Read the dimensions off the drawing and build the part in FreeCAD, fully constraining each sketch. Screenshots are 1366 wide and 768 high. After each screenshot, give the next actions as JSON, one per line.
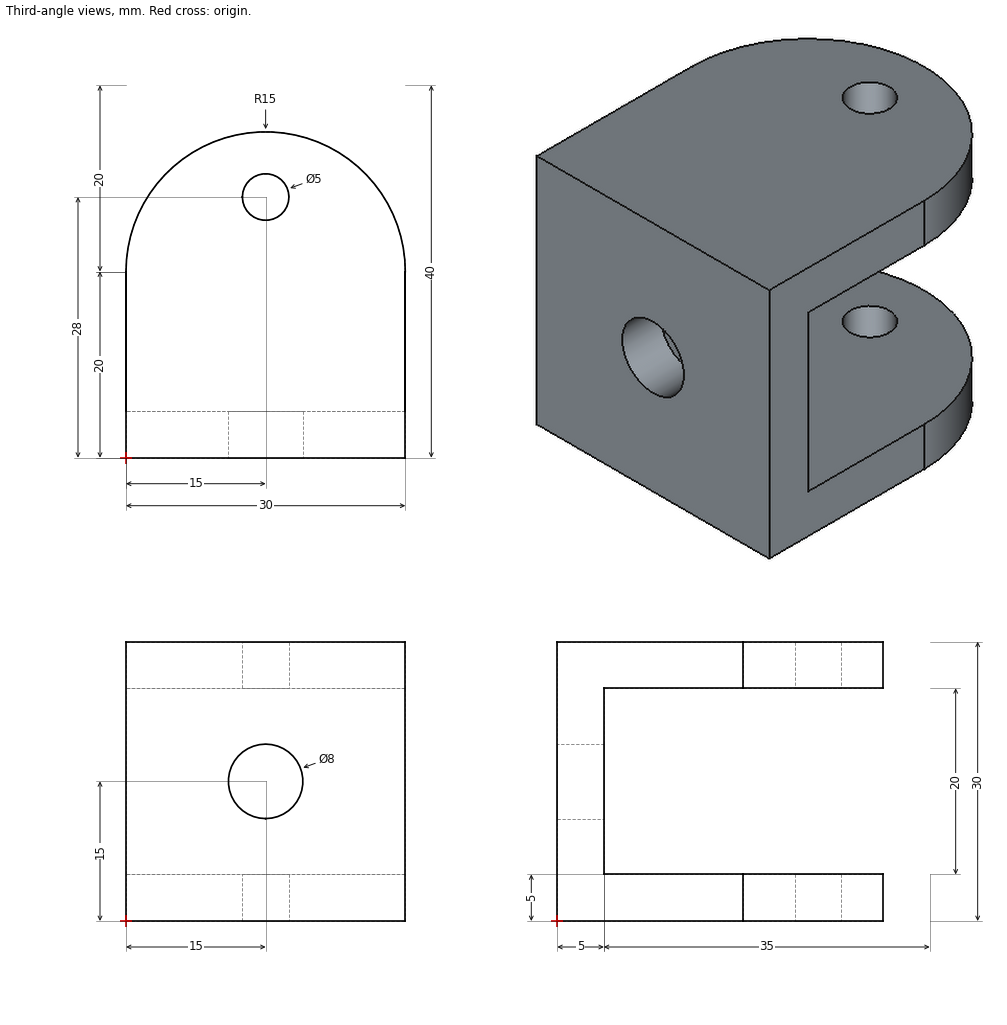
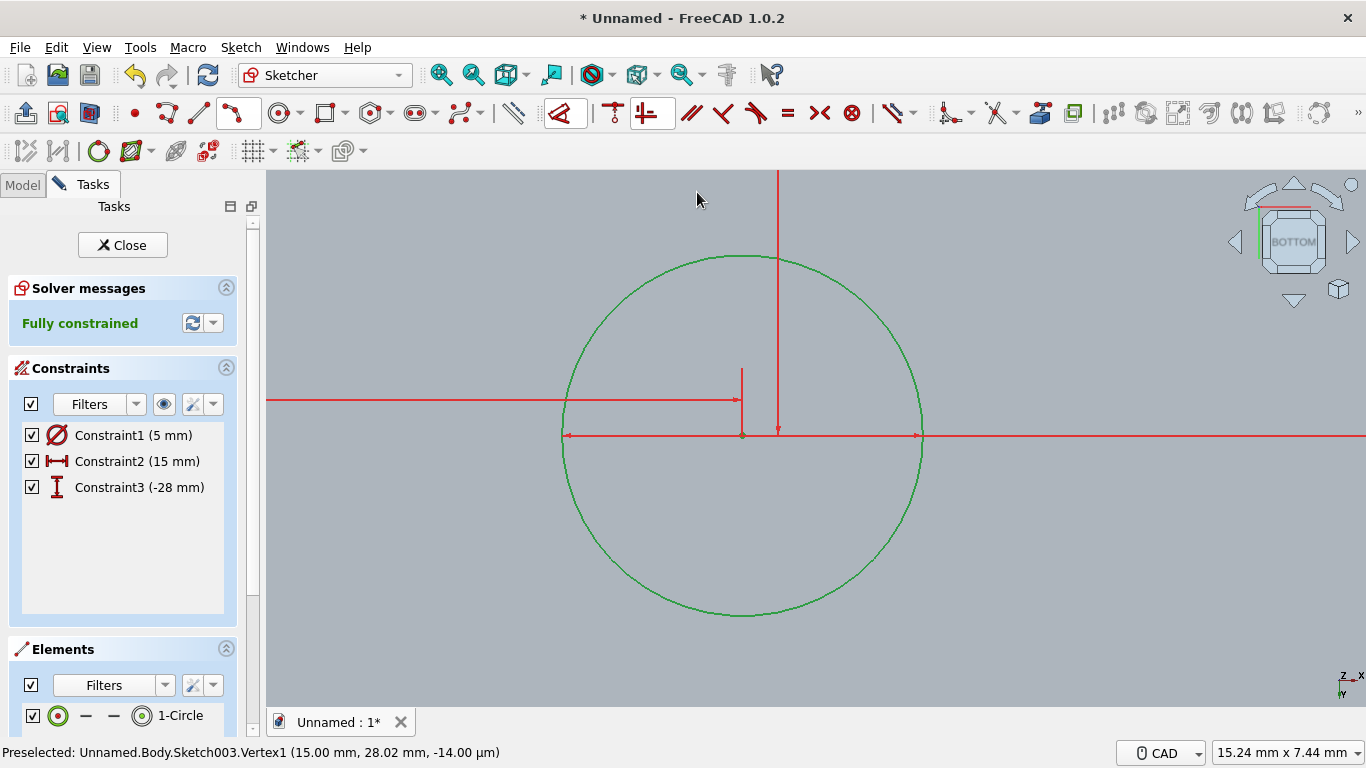
{"action": "left_click", "coordinate": [123, 245]}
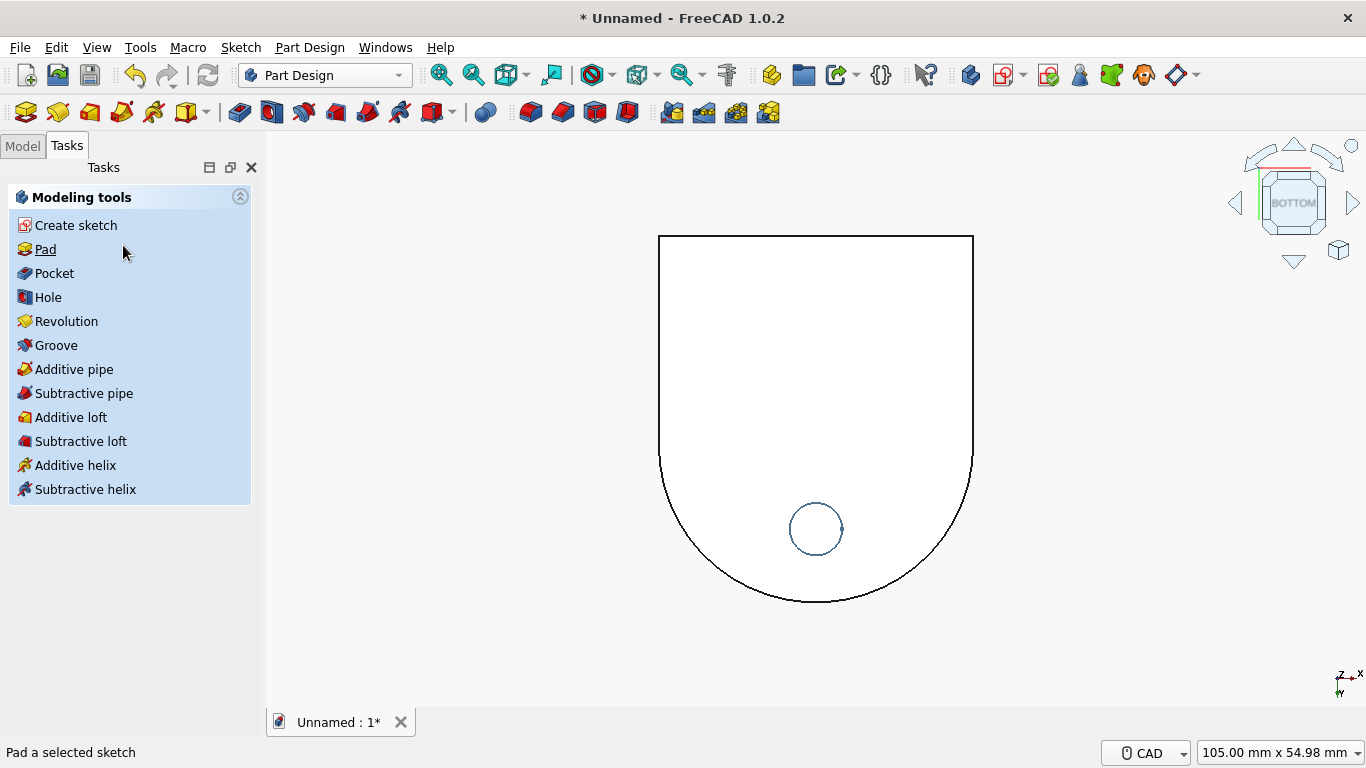
{"action": "left_click", "coordinate": [240, 112]}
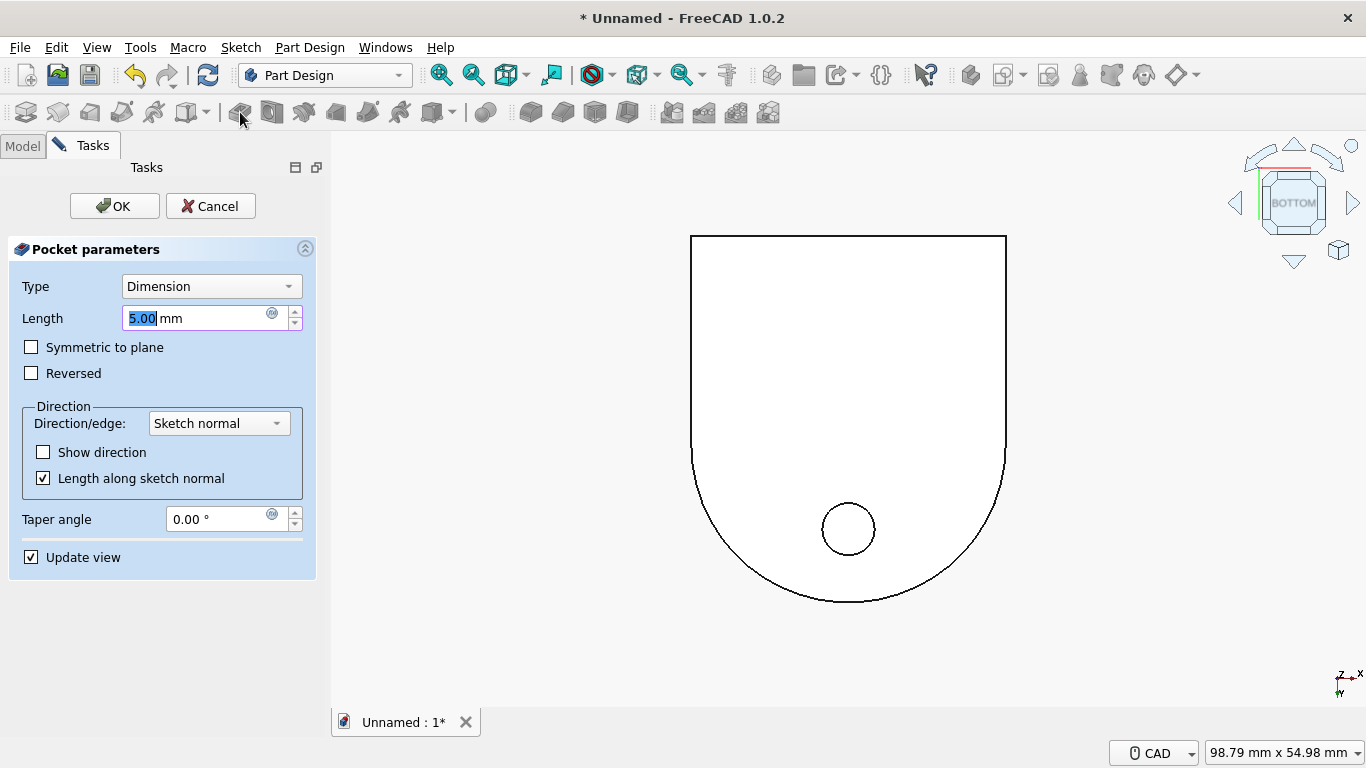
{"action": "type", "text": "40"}
{"action": "key", "text": "Tab"}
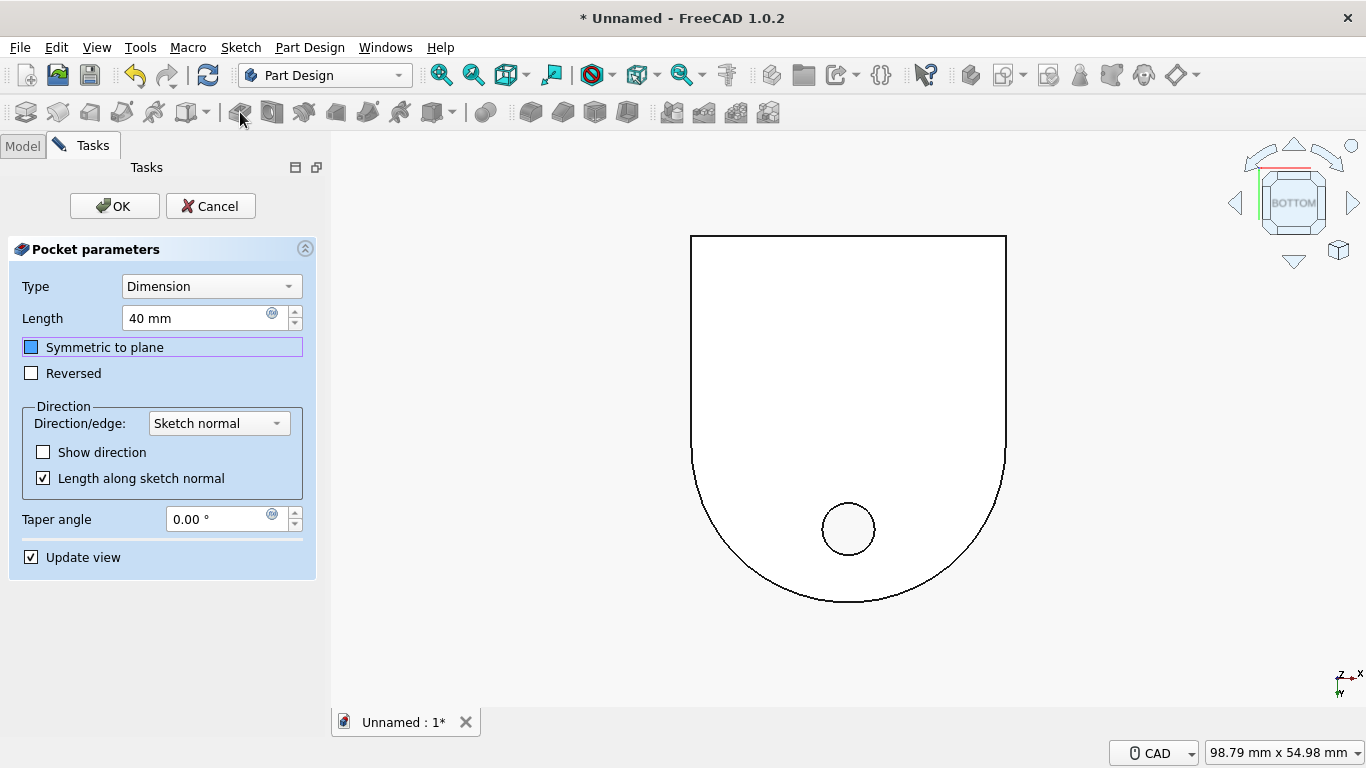
{"action": "left_click", "coordinate": [115, 206]}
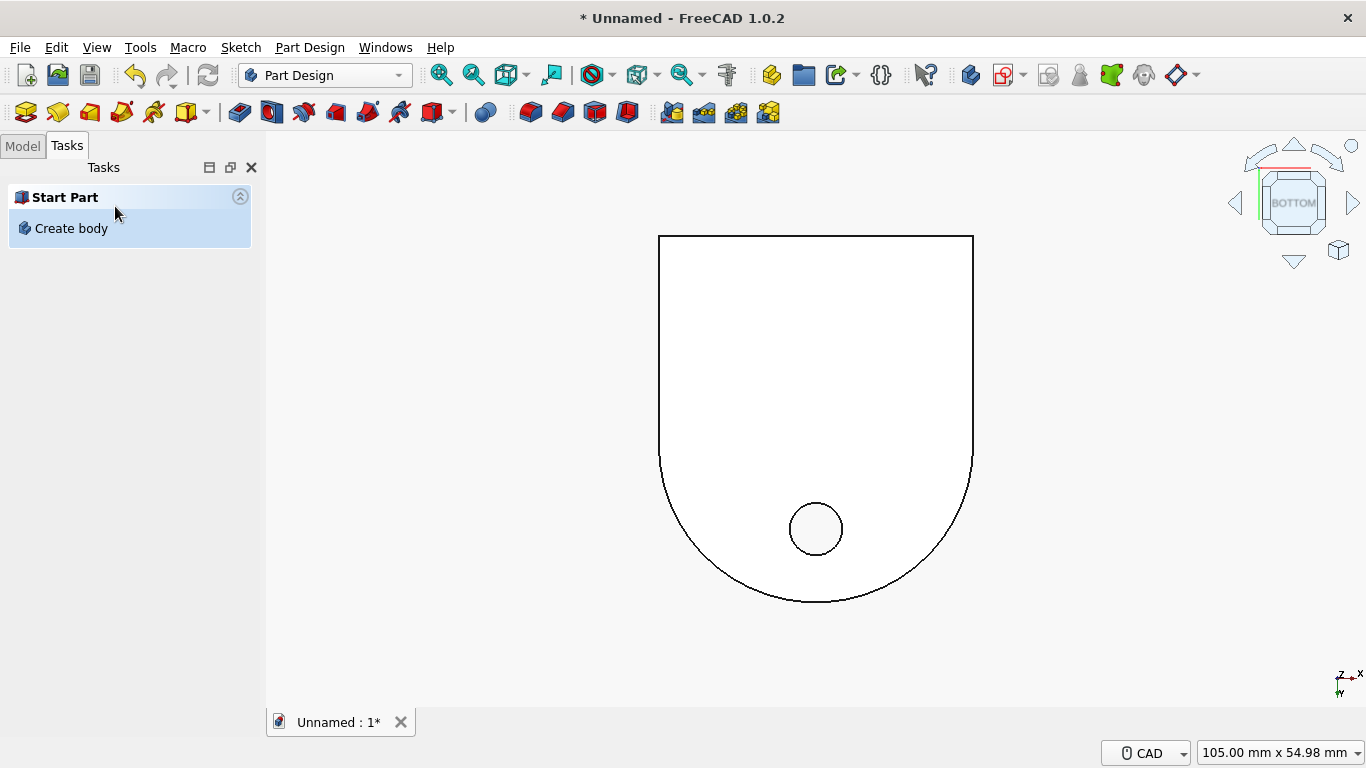
{"action": "left_click", "coordinate": [1004, 76]}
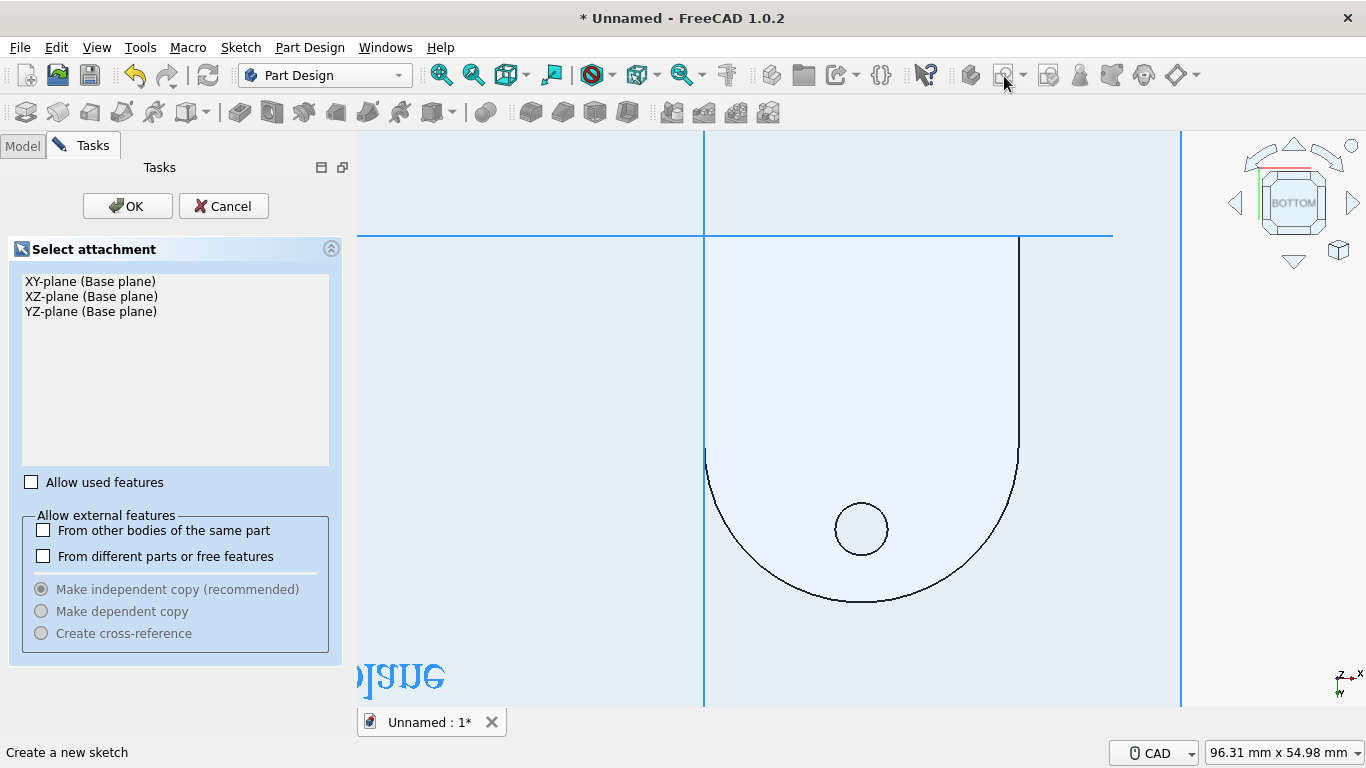
{"action": "left_click", "coordinate": [82, 296]}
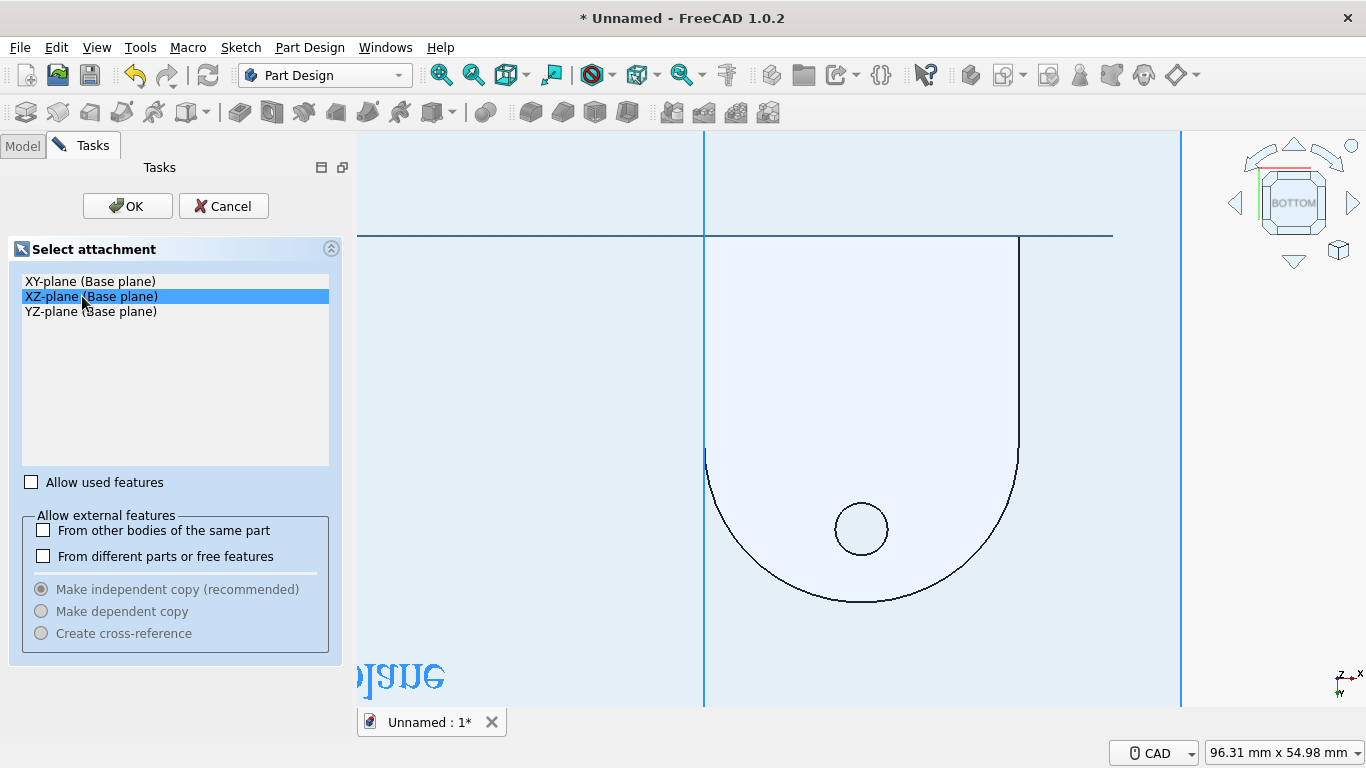
{"action": "left_click", "coordinate": [128, 206]}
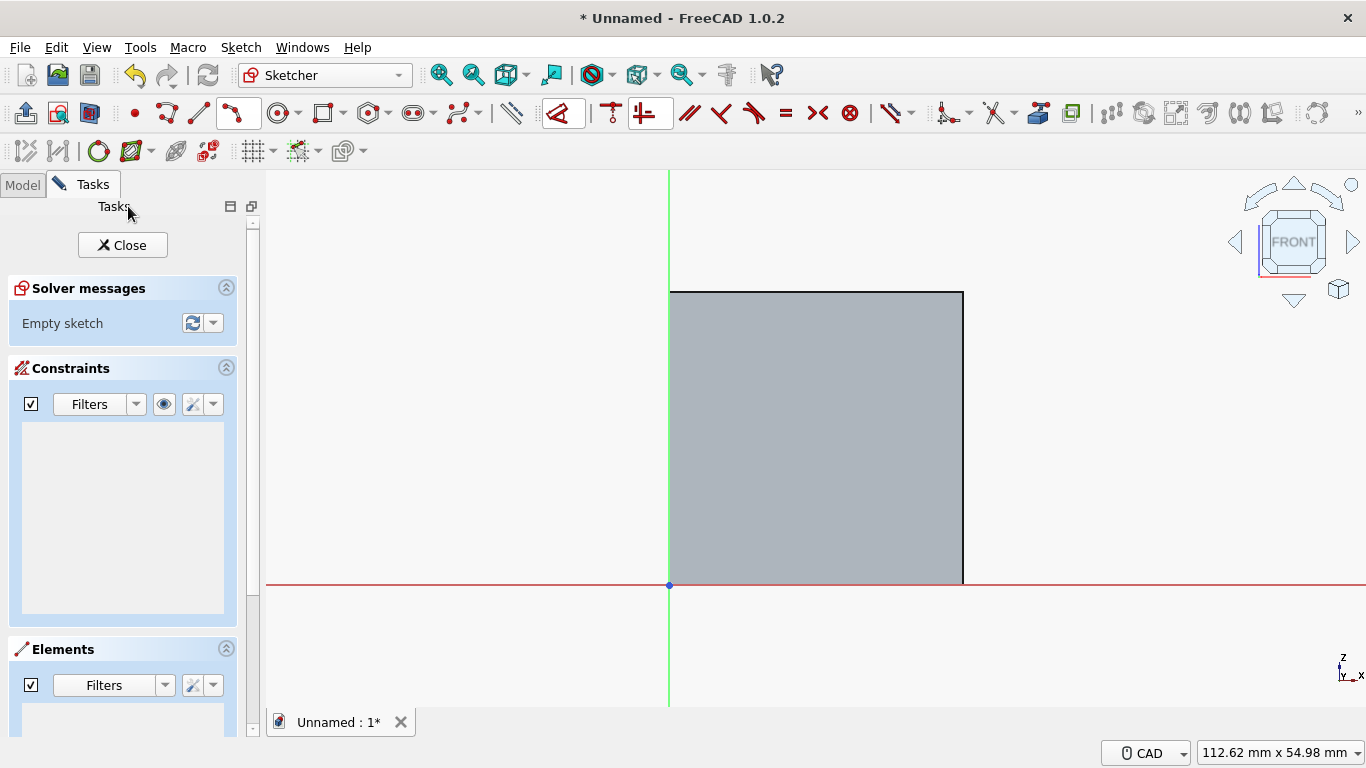
{"action": "scroll", "coordinate": [780, 558], "scroll_direction": "up", "scroll_amount": 3}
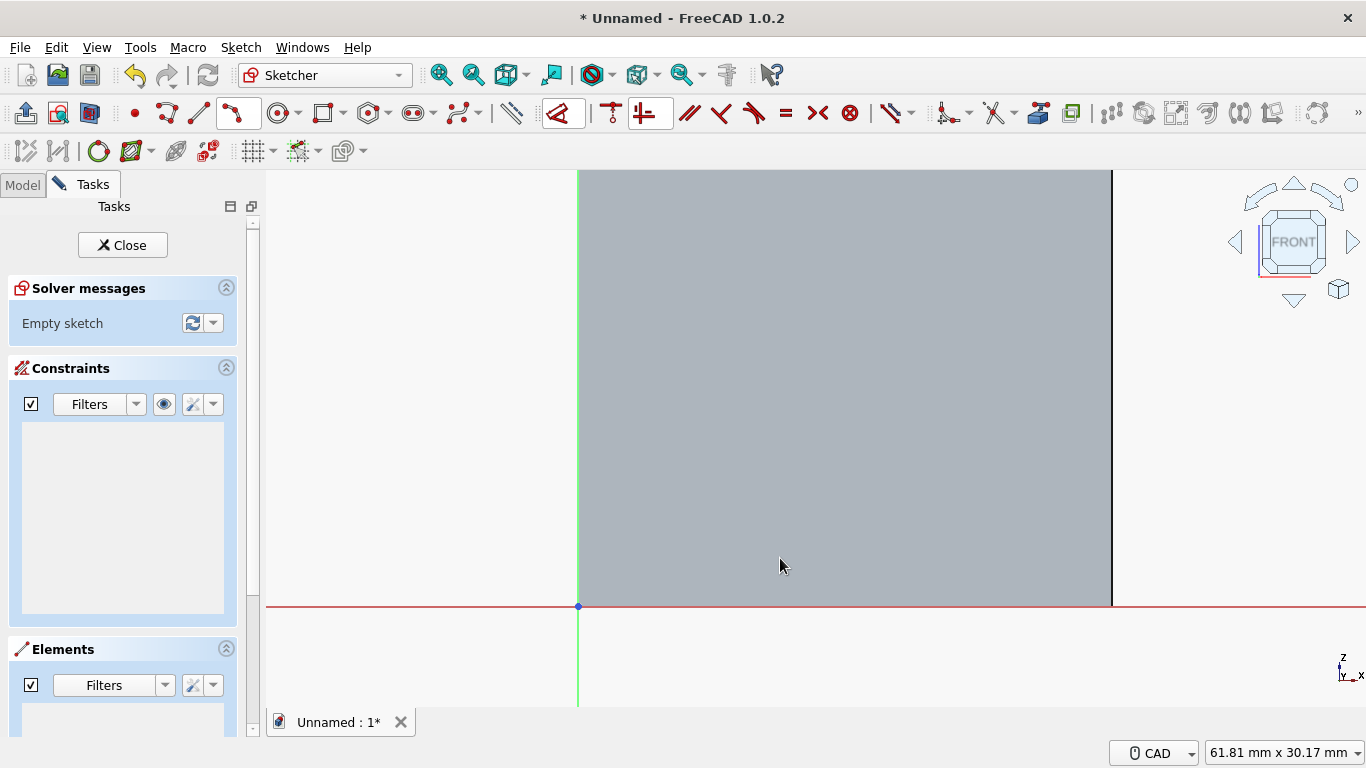
{"action": "left_click", "coordinate": [278, 114]}